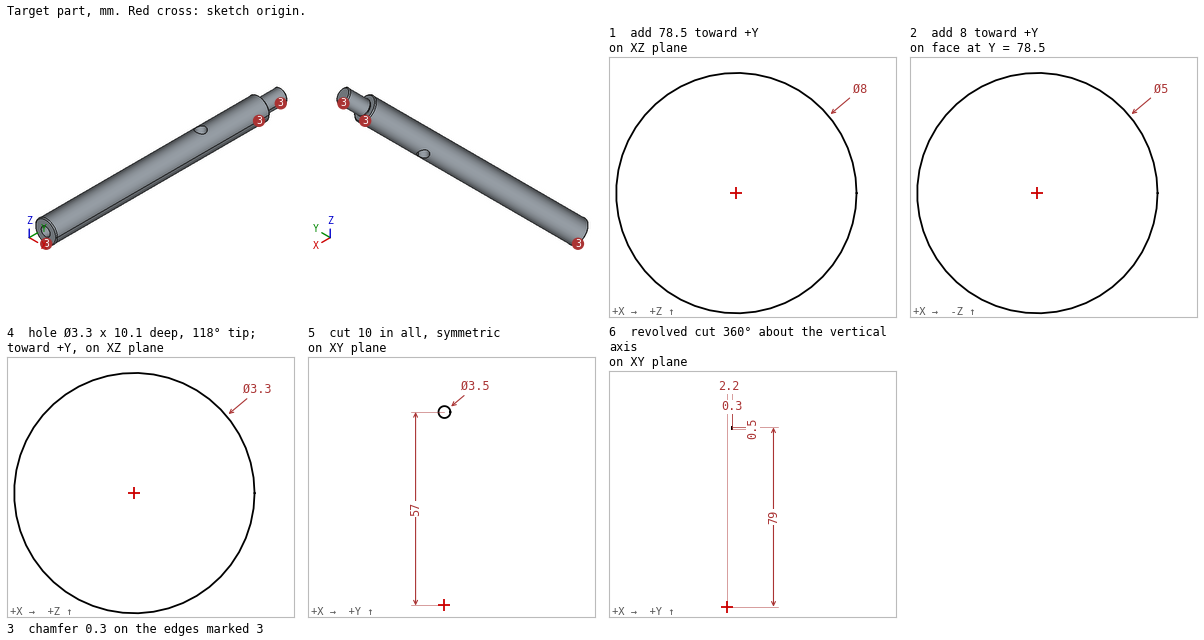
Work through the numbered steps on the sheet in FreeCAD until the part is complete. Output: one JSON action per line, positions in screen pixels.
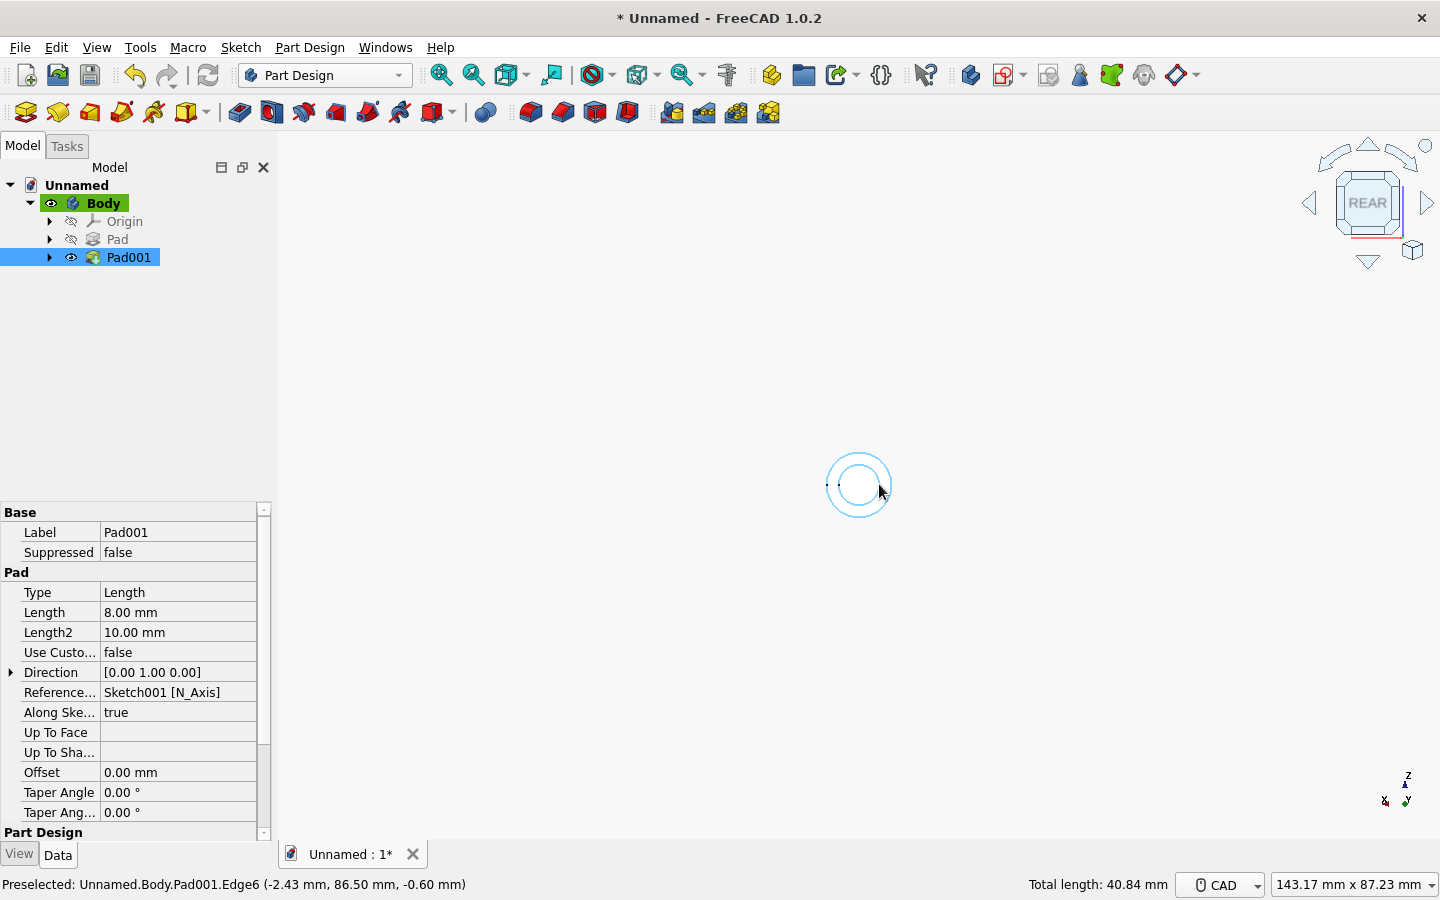
{"action": "key", "text": "0"}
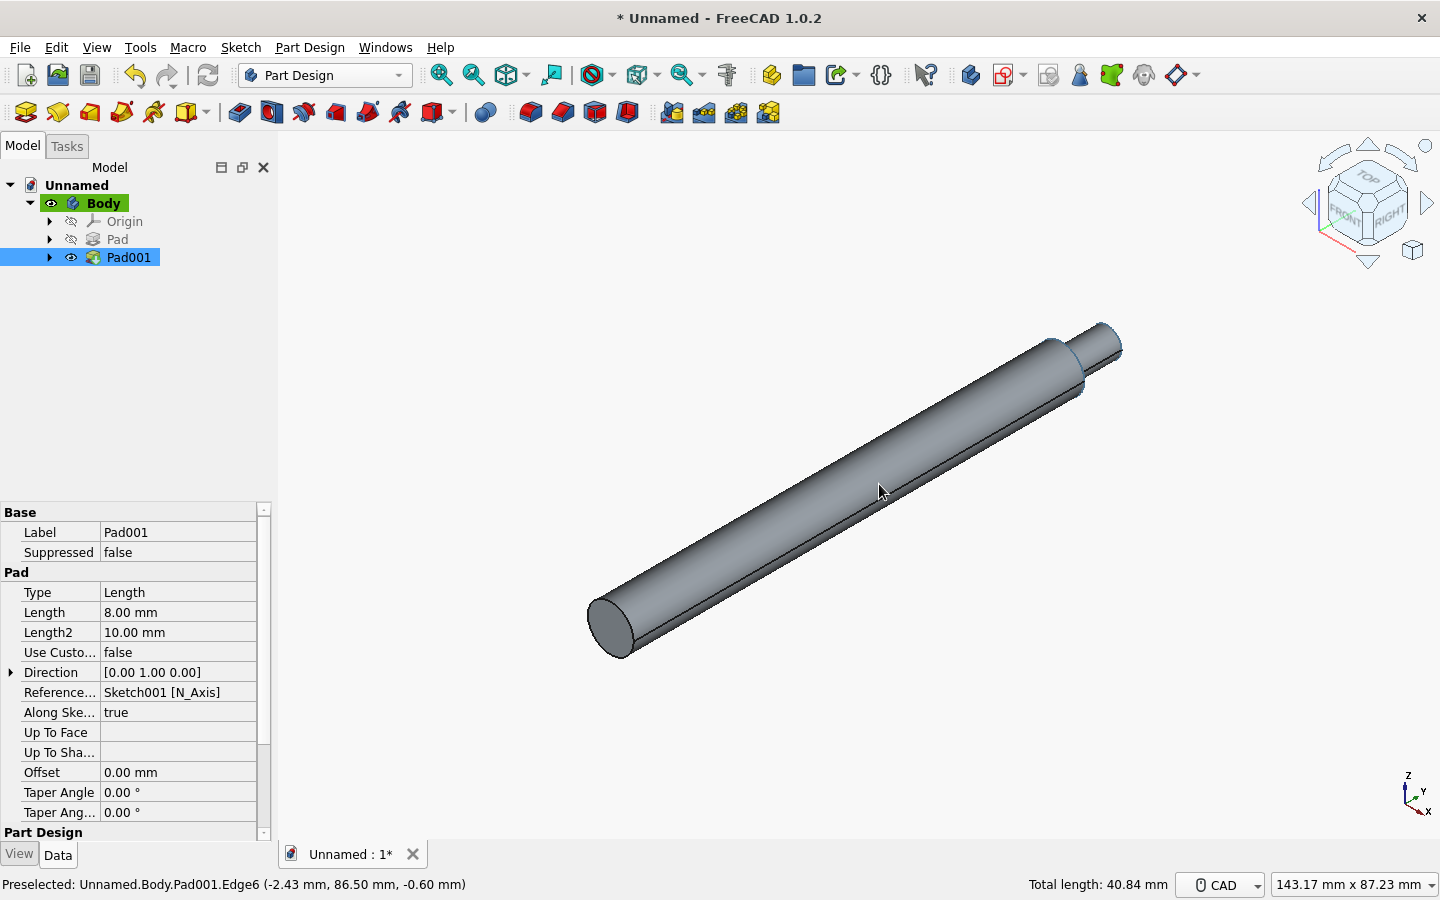
{"action": "left_click", "coordinate": [592, 601], "text": "ctrl"}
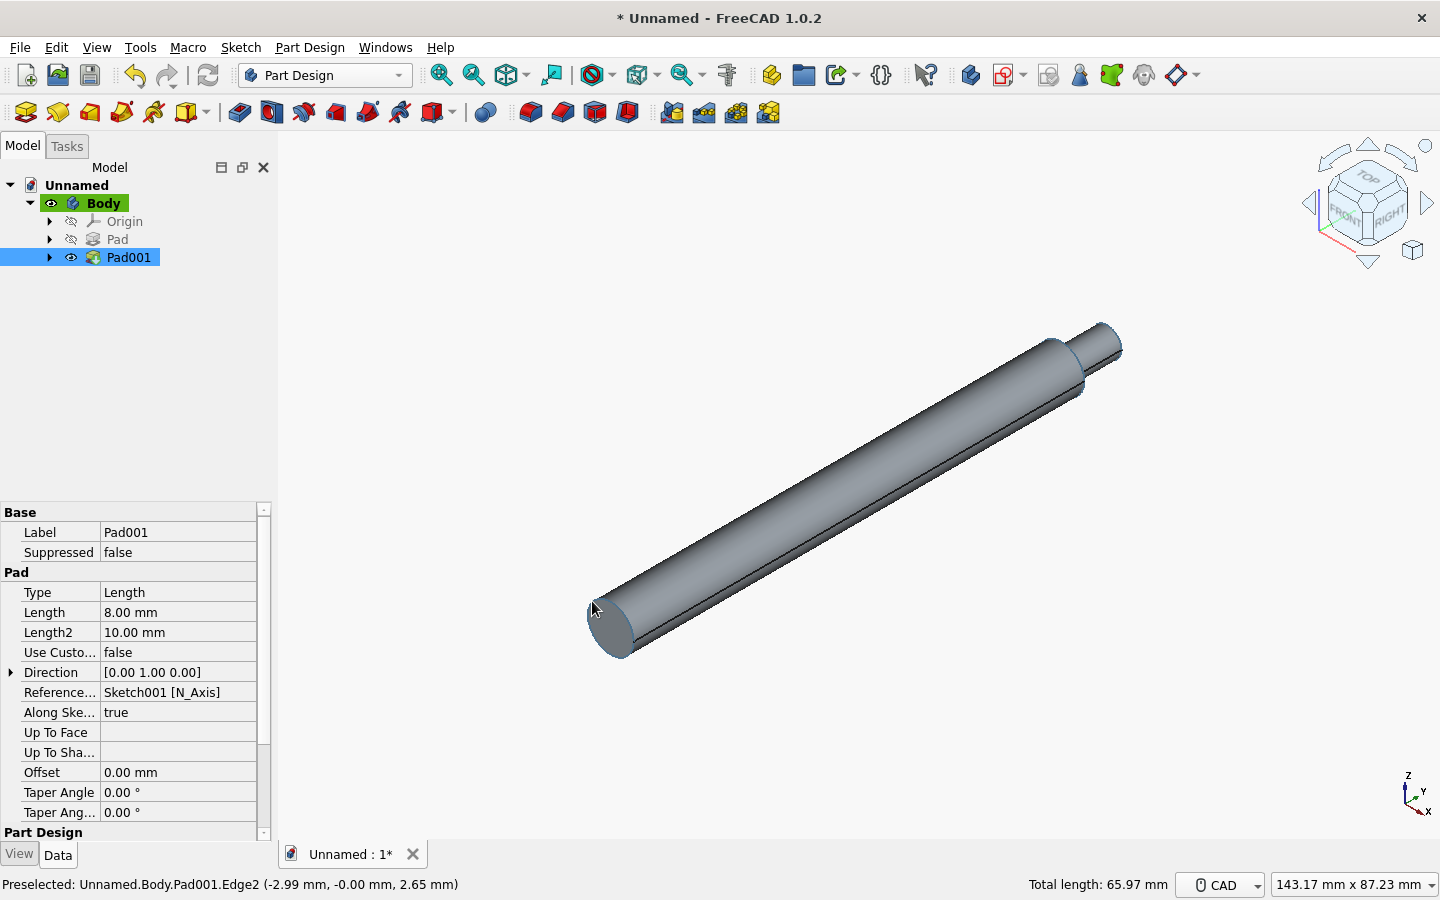
{"action": "left_click", "coordinate": [564, 112]}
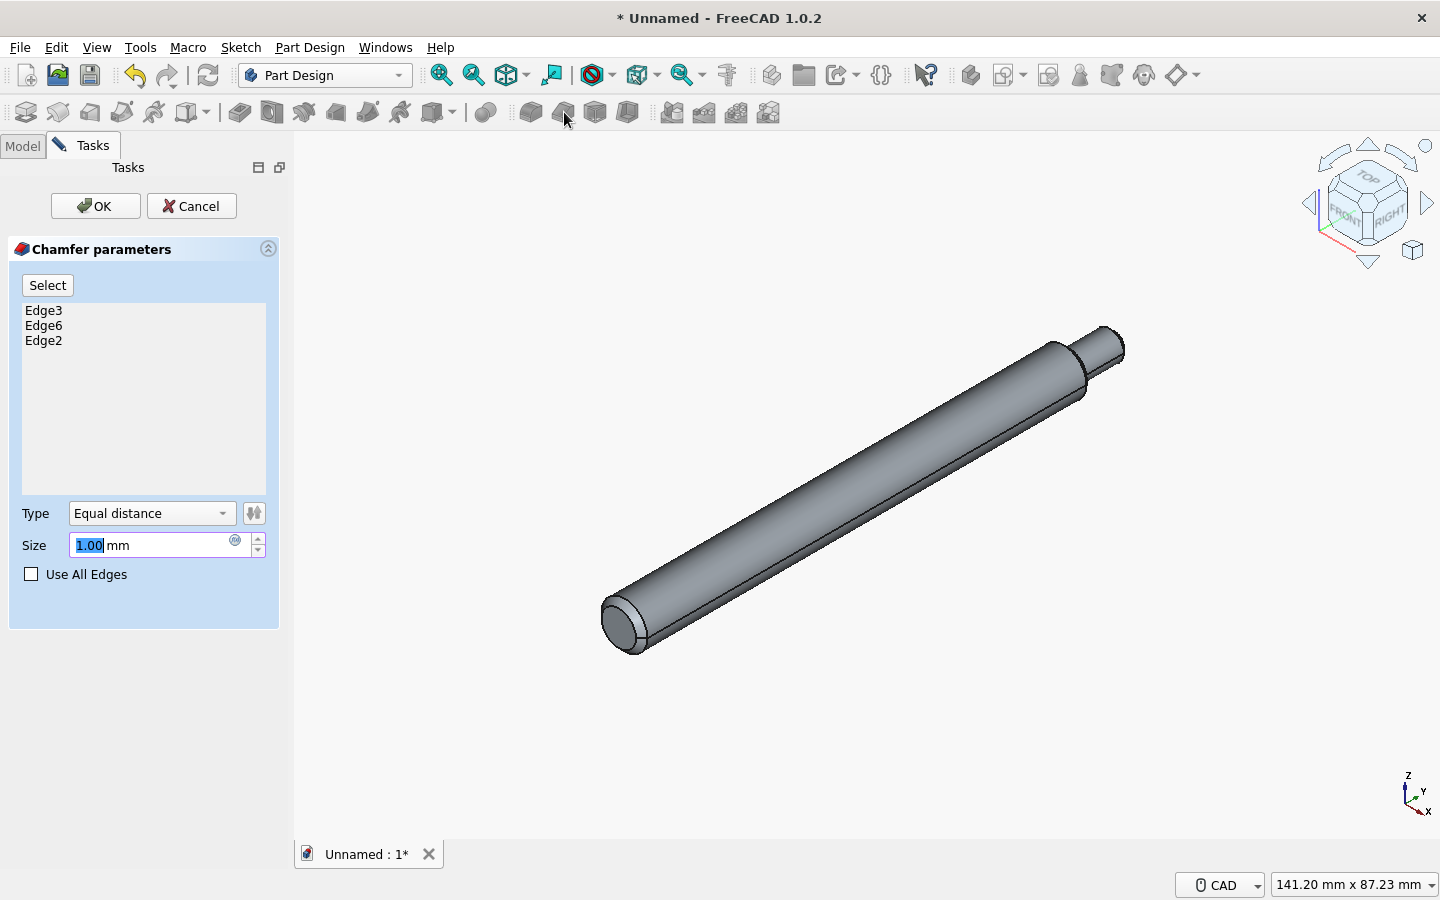
{"action": "type", "text": "0.3"}
{"action": "key", "text": "Tab"}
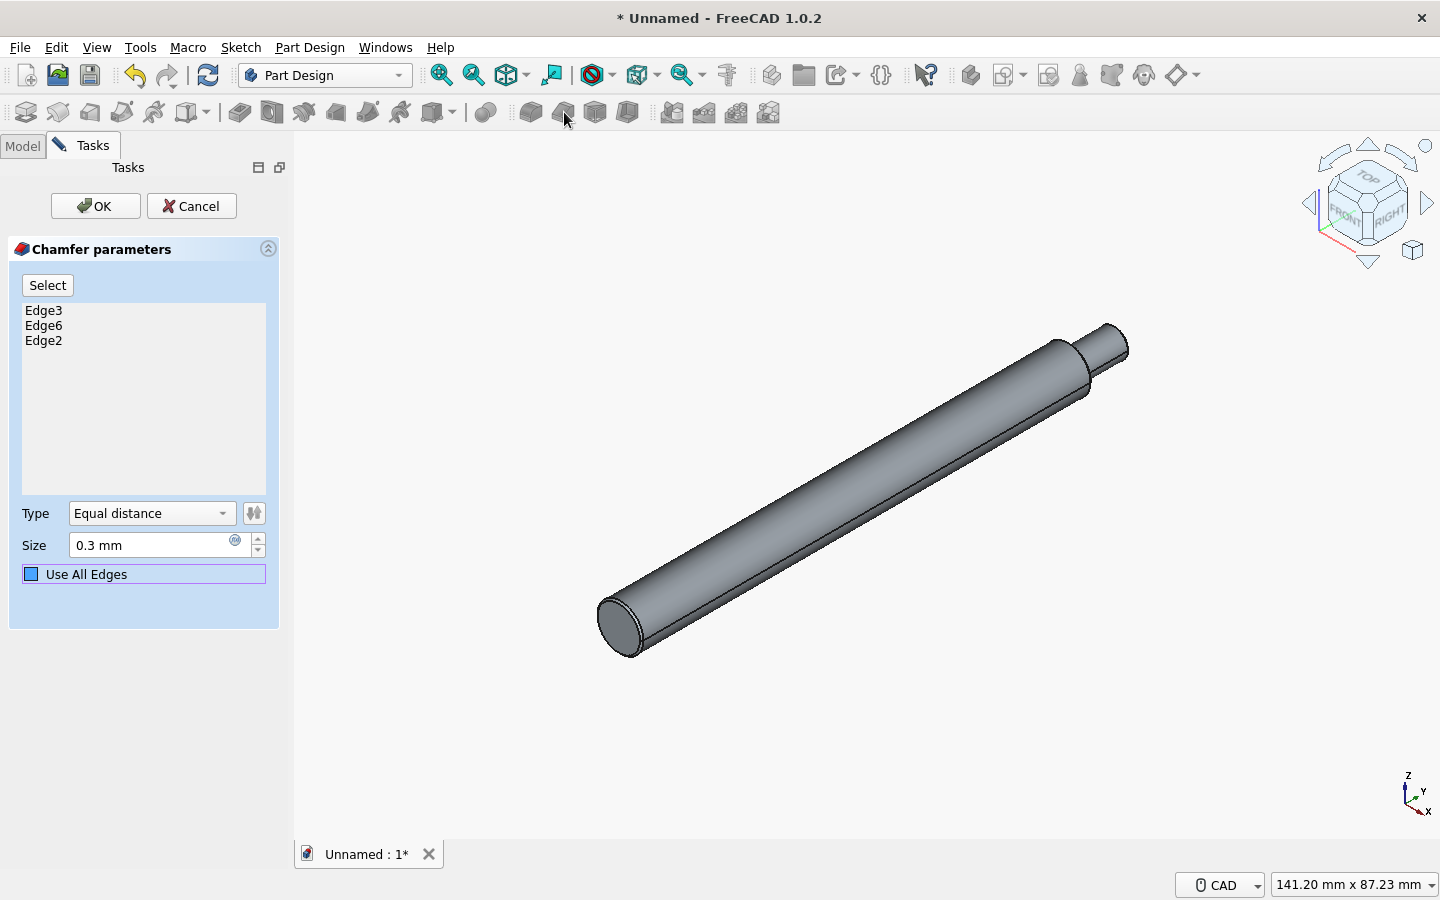
{"action": "left_click", "coordinate": [96, 206]}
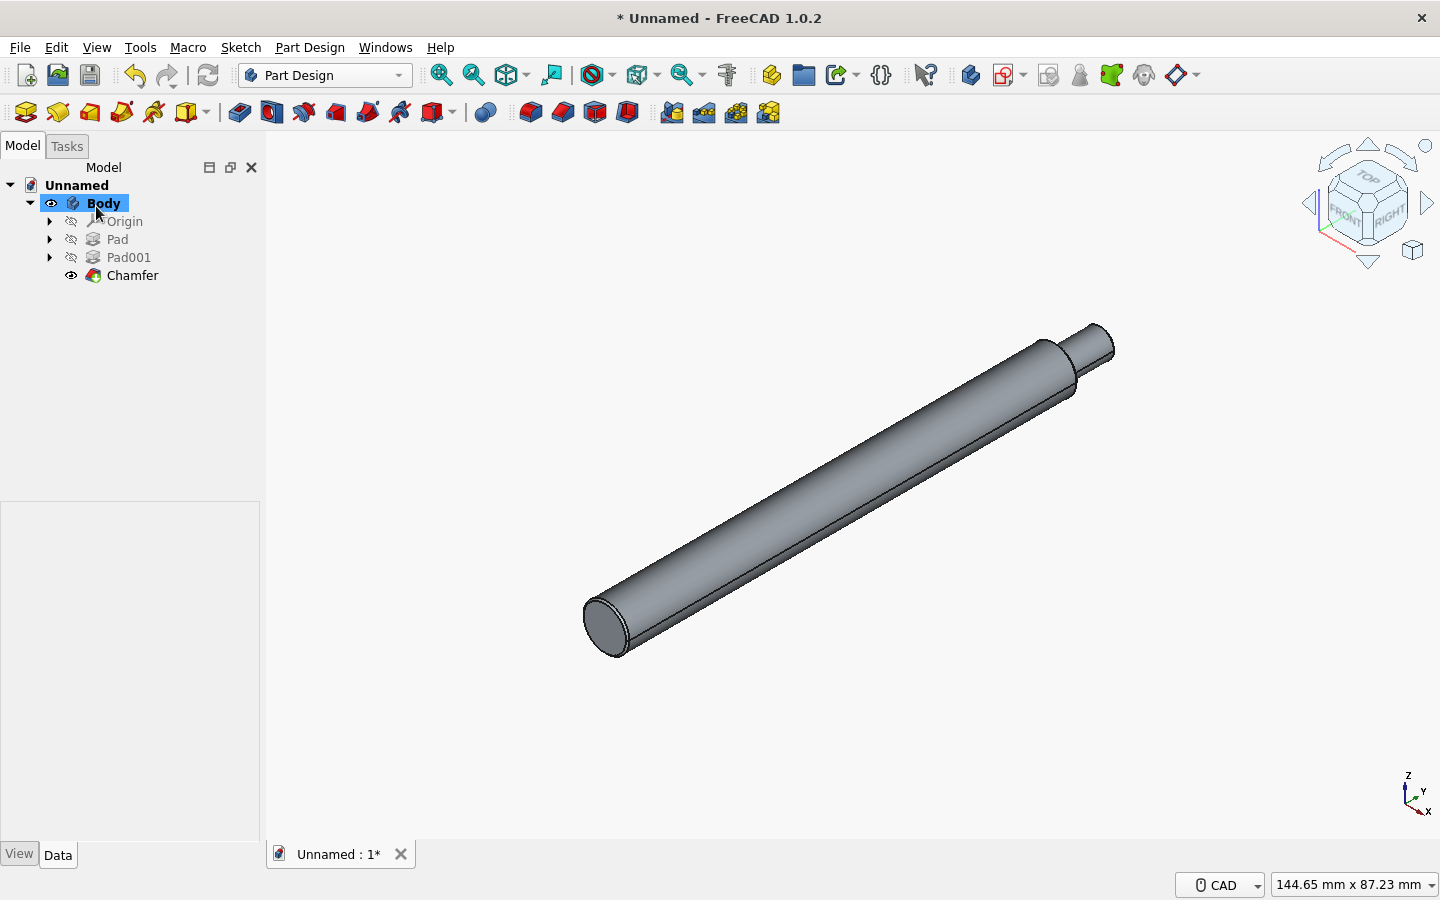
{"action": "left_click", "coordinate": [1004, 76]}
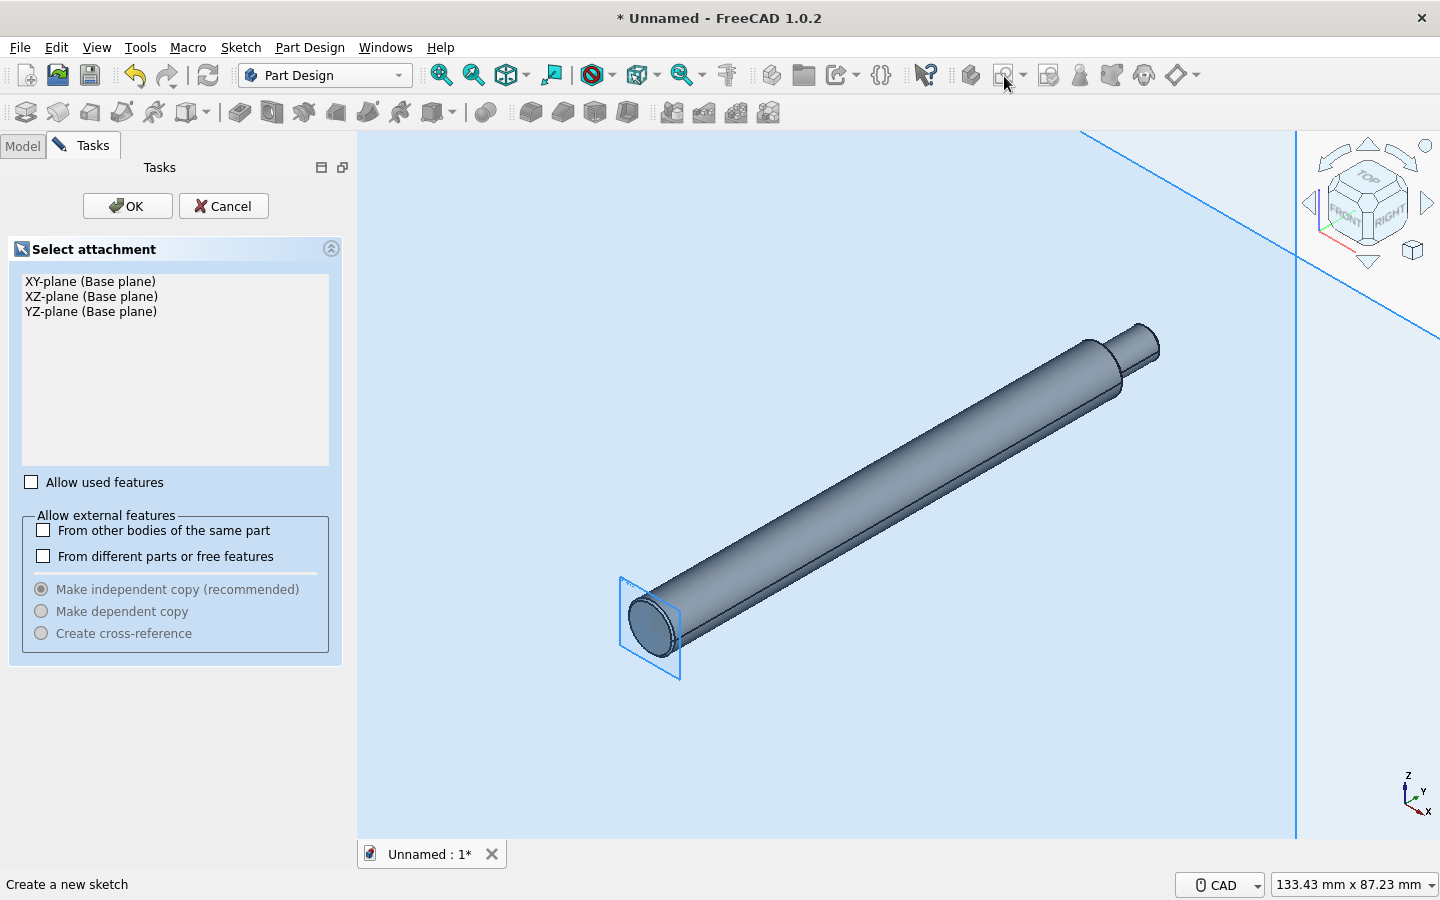
{"action": "left_click", "coordinate": [82, 296]}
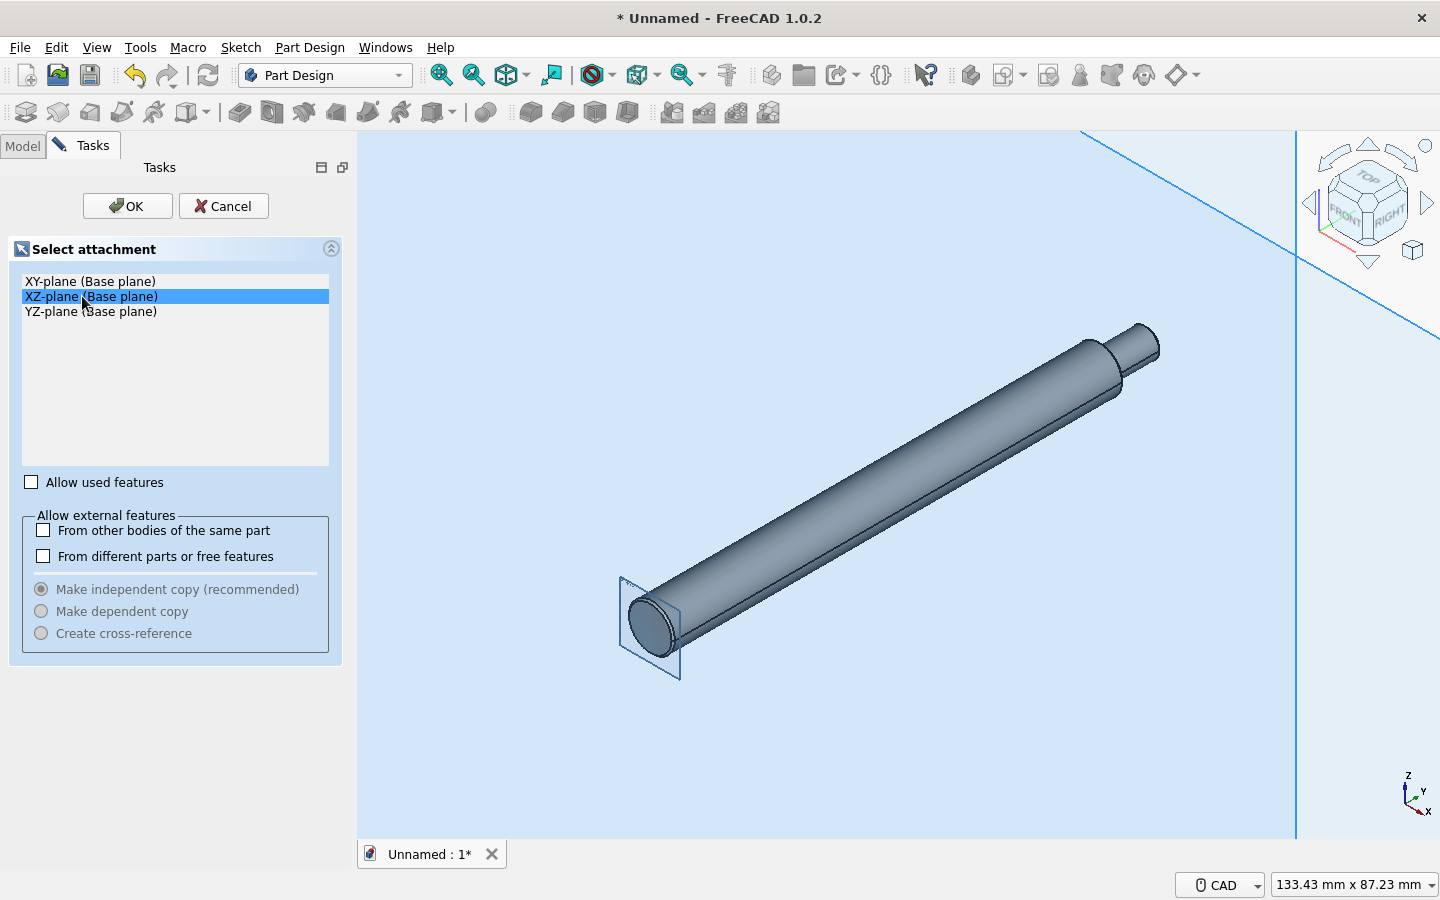
{"action": "left_click", "coordinate": [128, 206]}